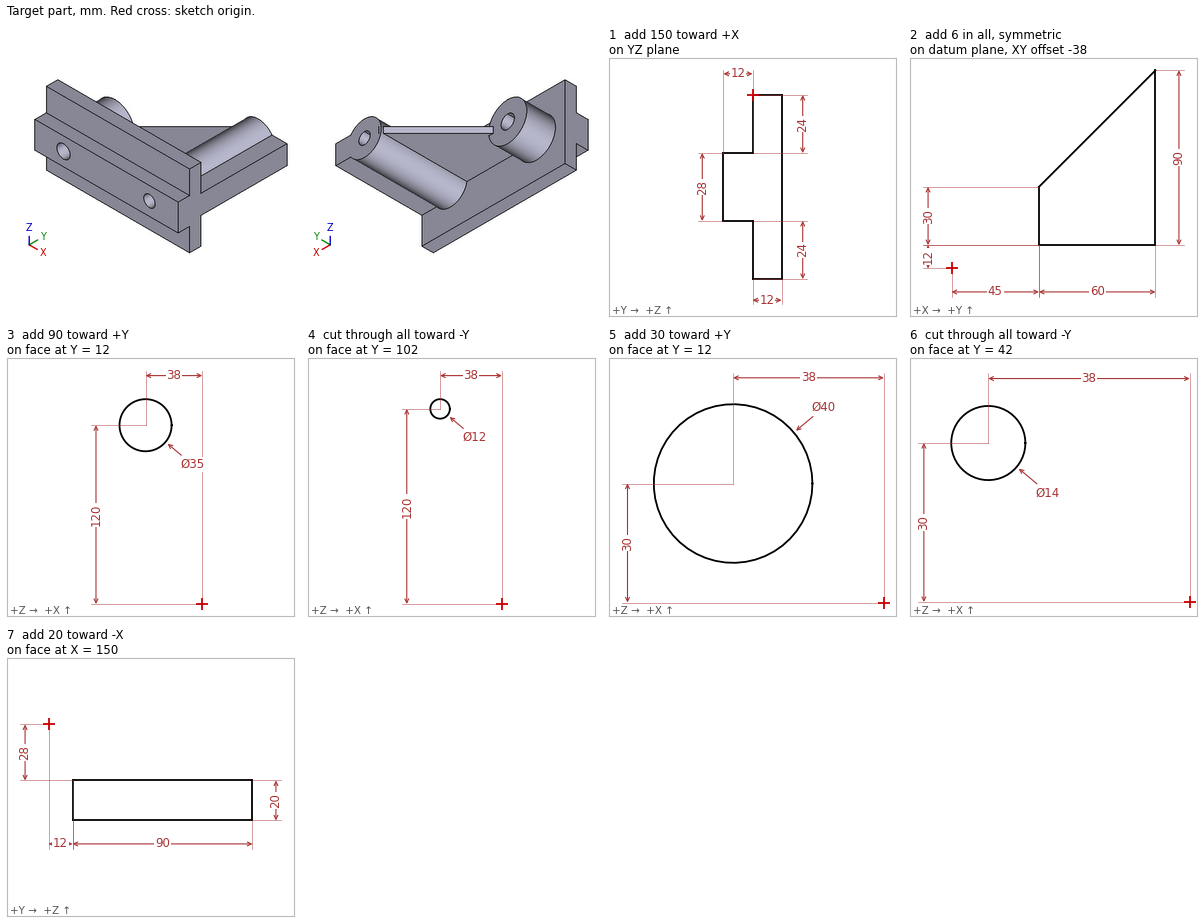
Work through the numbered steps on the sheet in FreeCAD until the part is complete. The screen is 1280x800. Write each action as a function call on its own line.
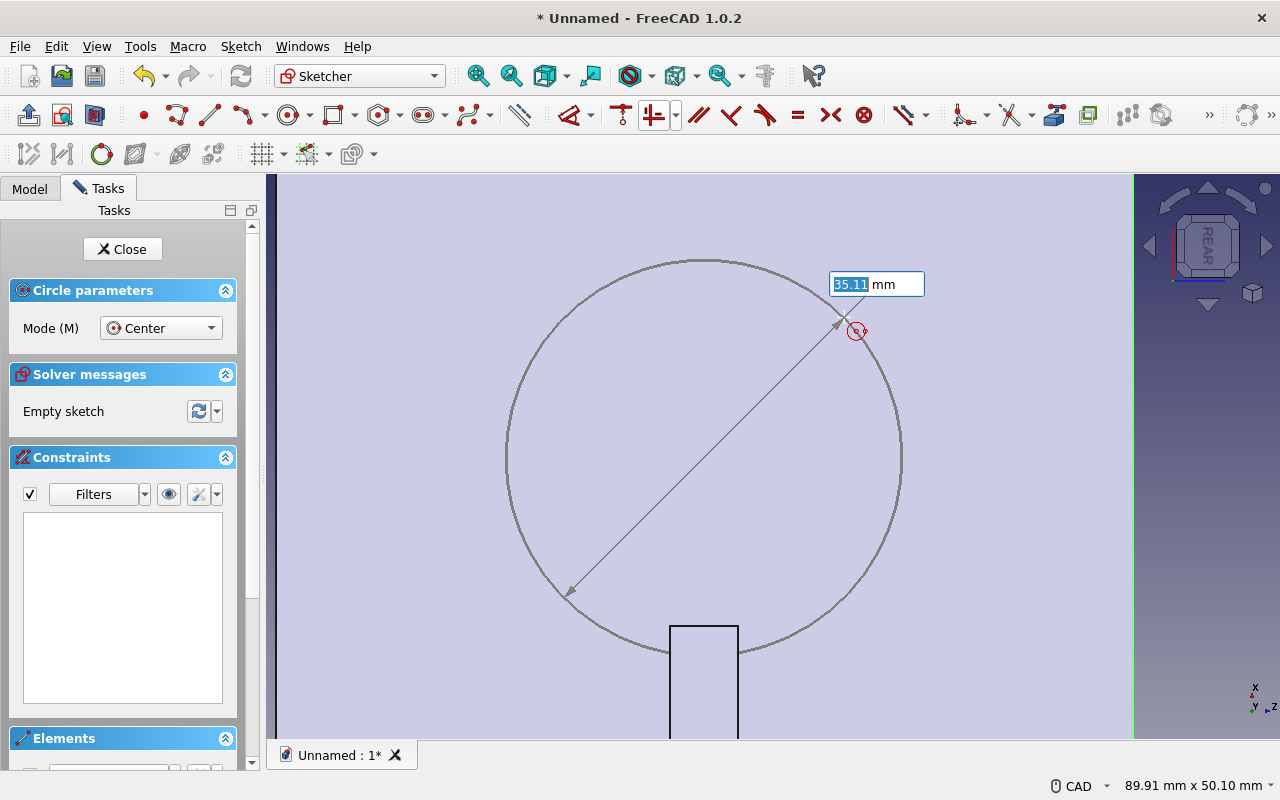
text(35)
key(Return)
key(Escape)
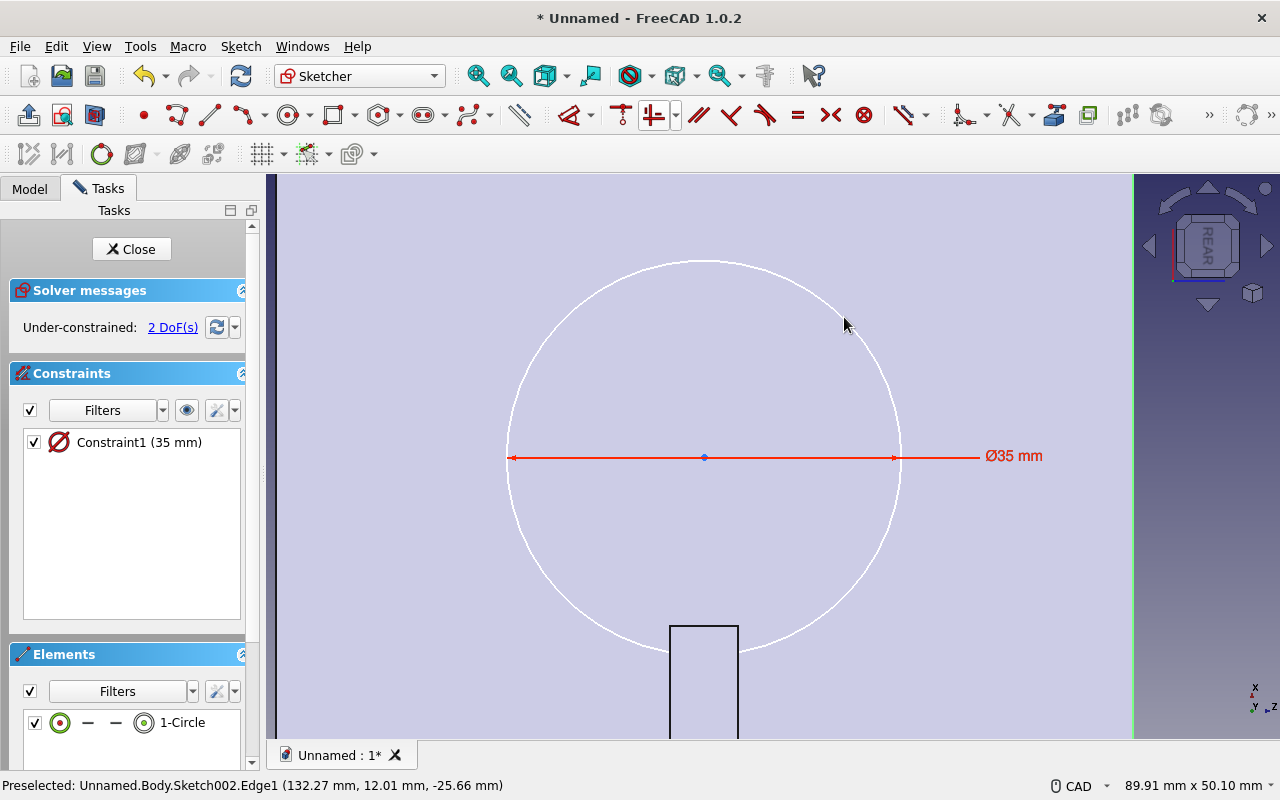
click(568, 116)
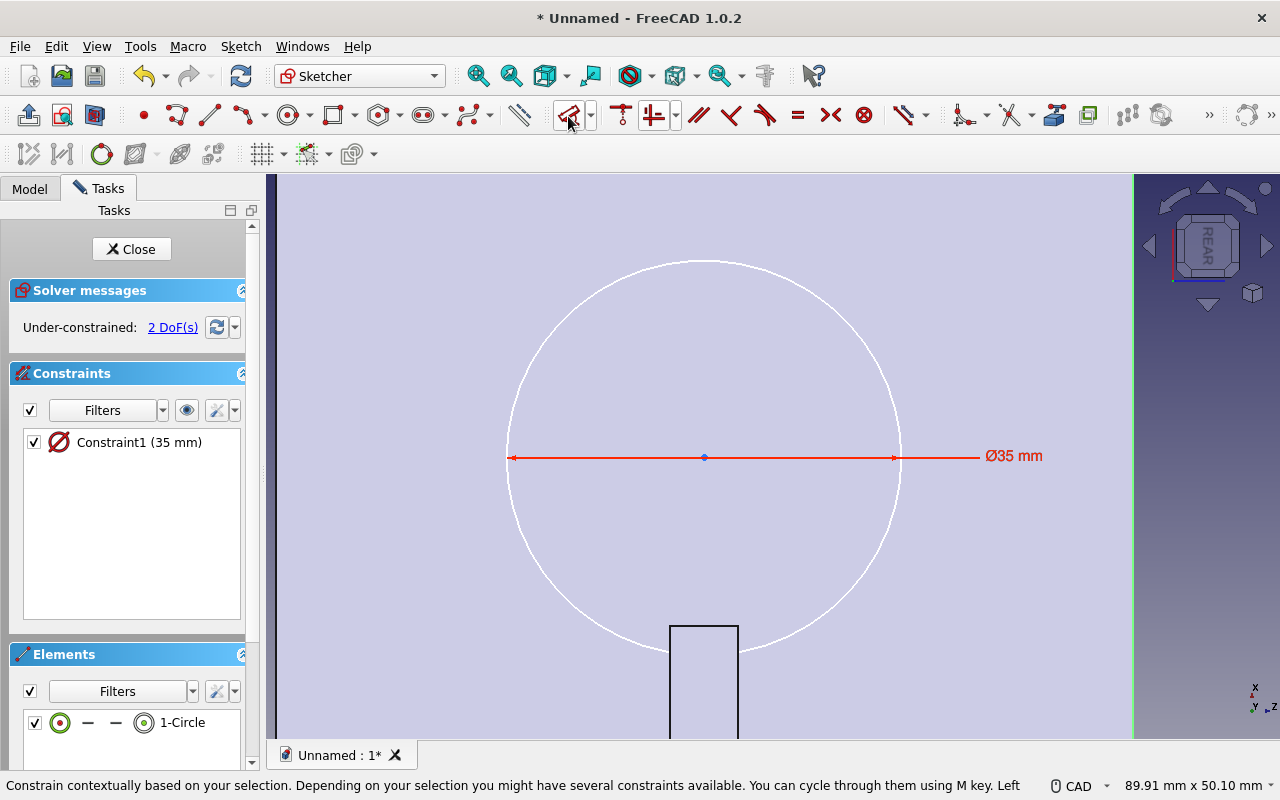
click(704, 458)
click(815, 424)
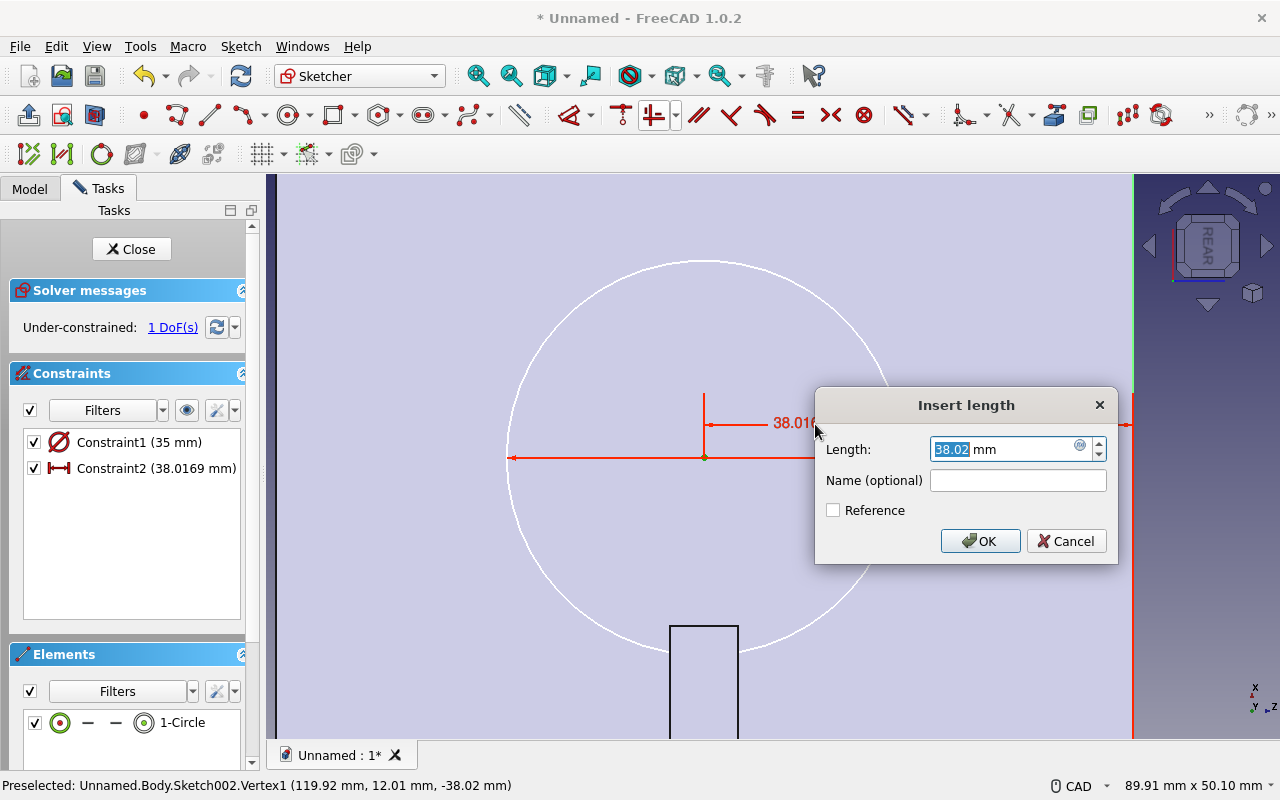
text(38)
key(Return)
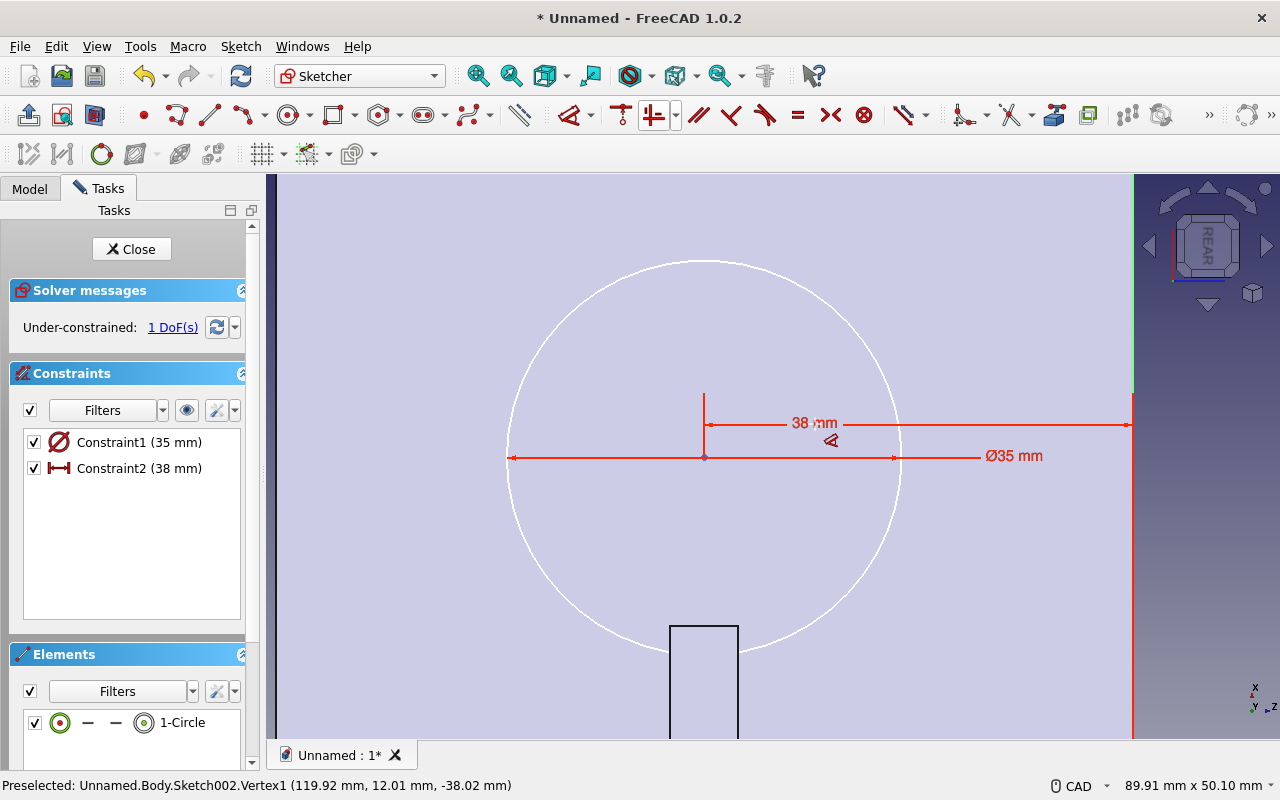
click(704, 458)
click(670, 585)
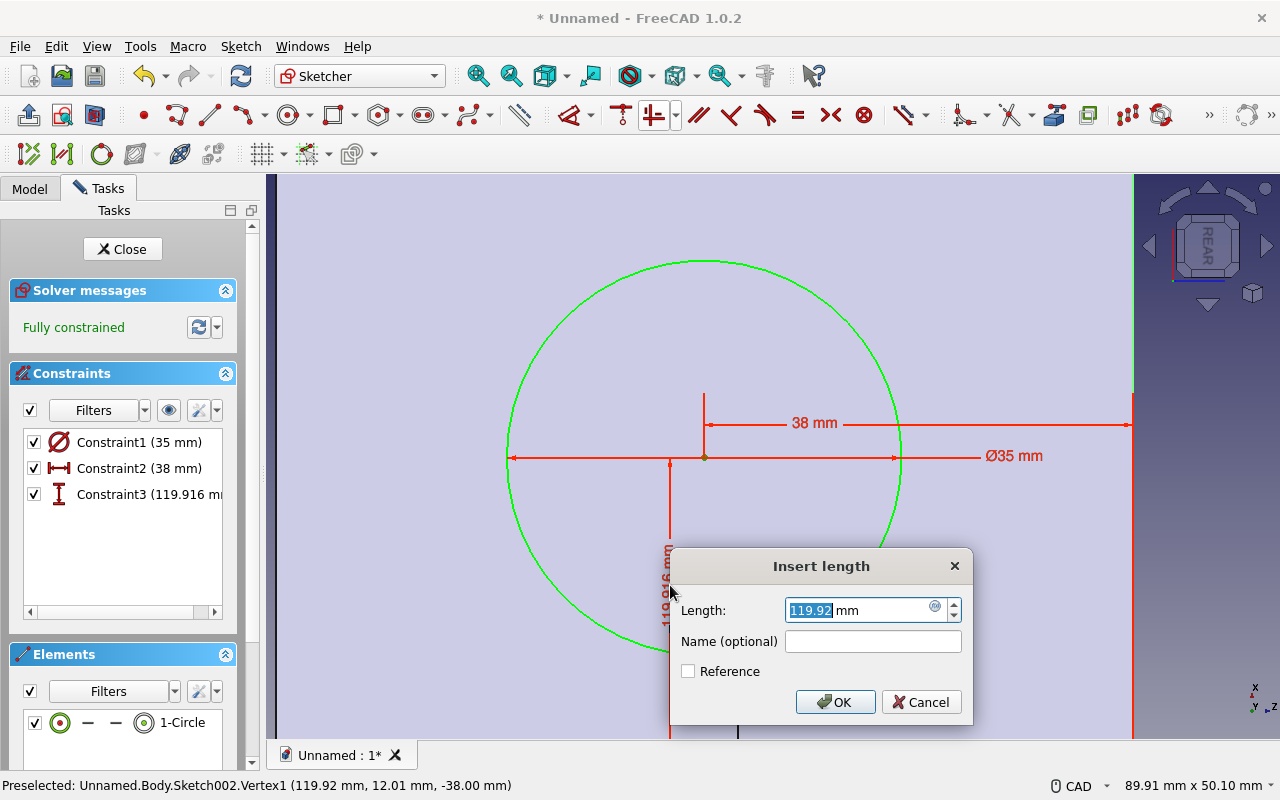
text(120)
key(Return)
key(Escape)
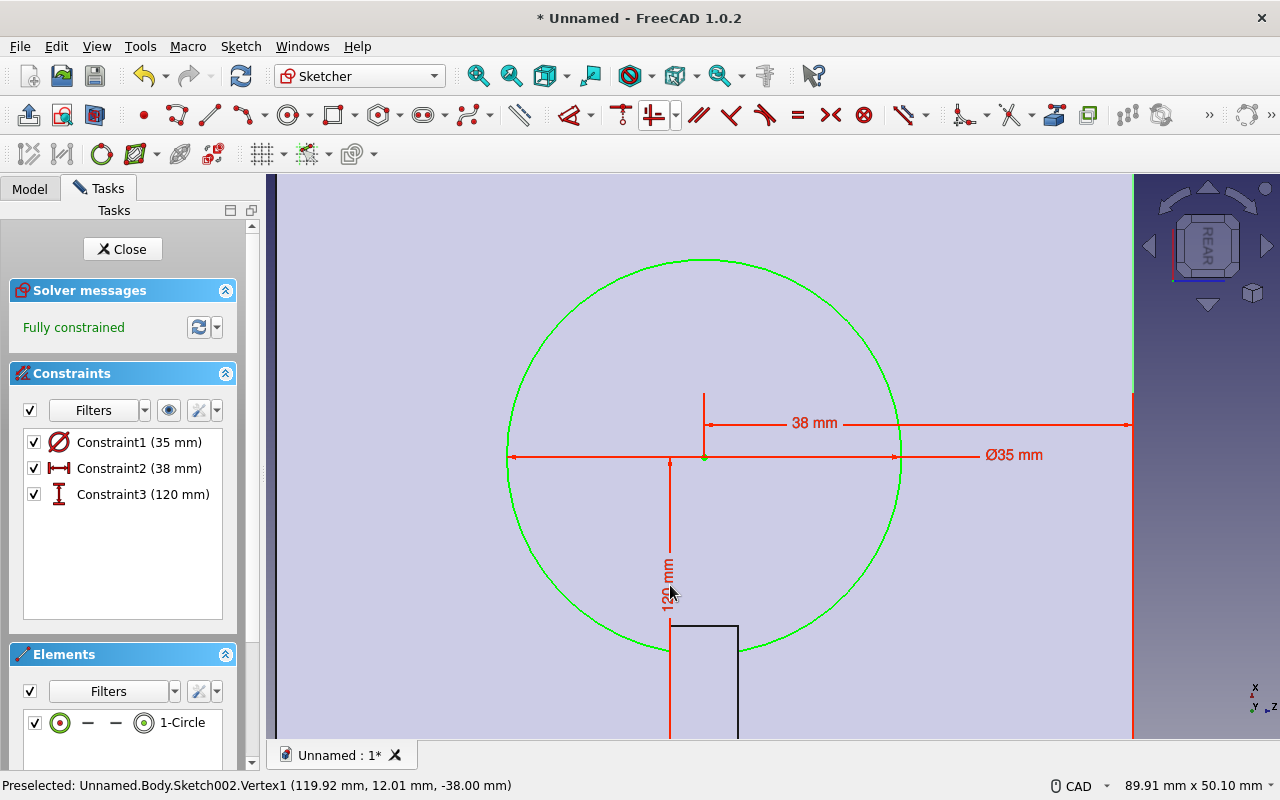
click(123, 249)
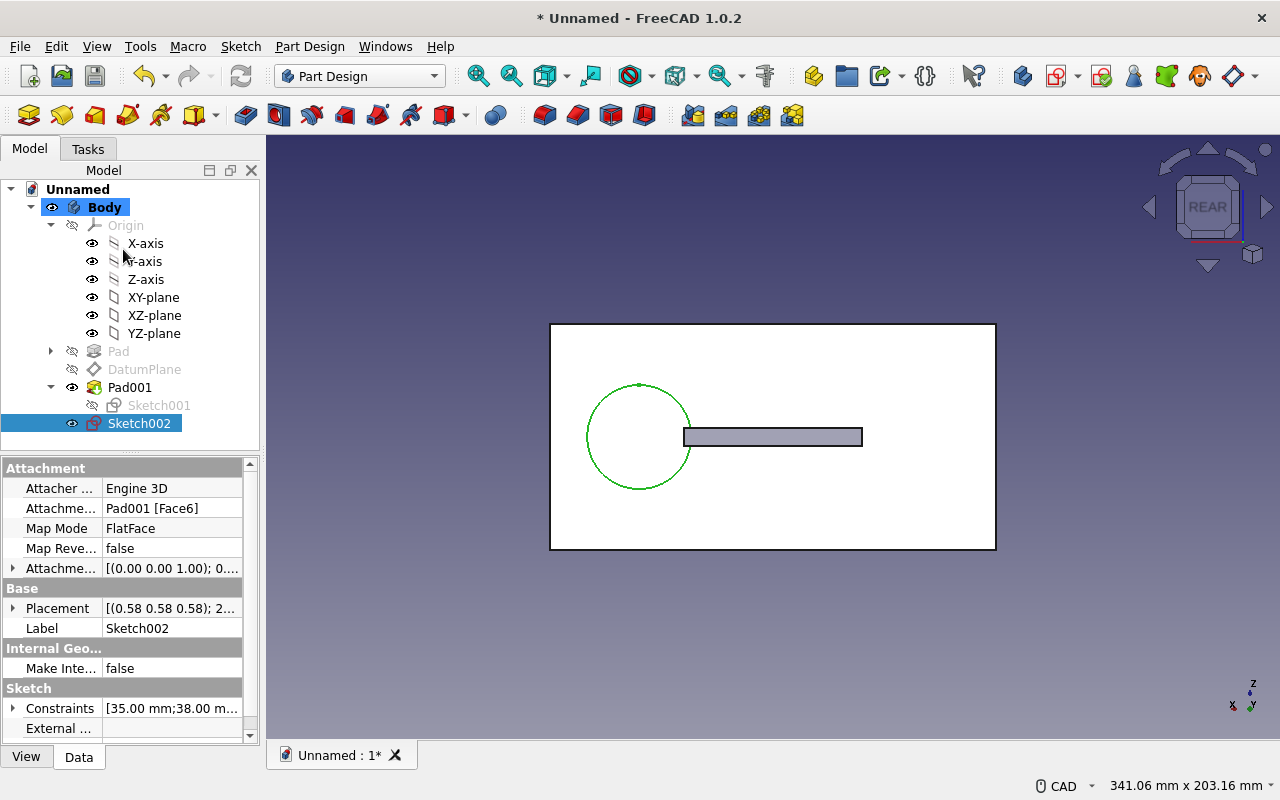
click(29, 116)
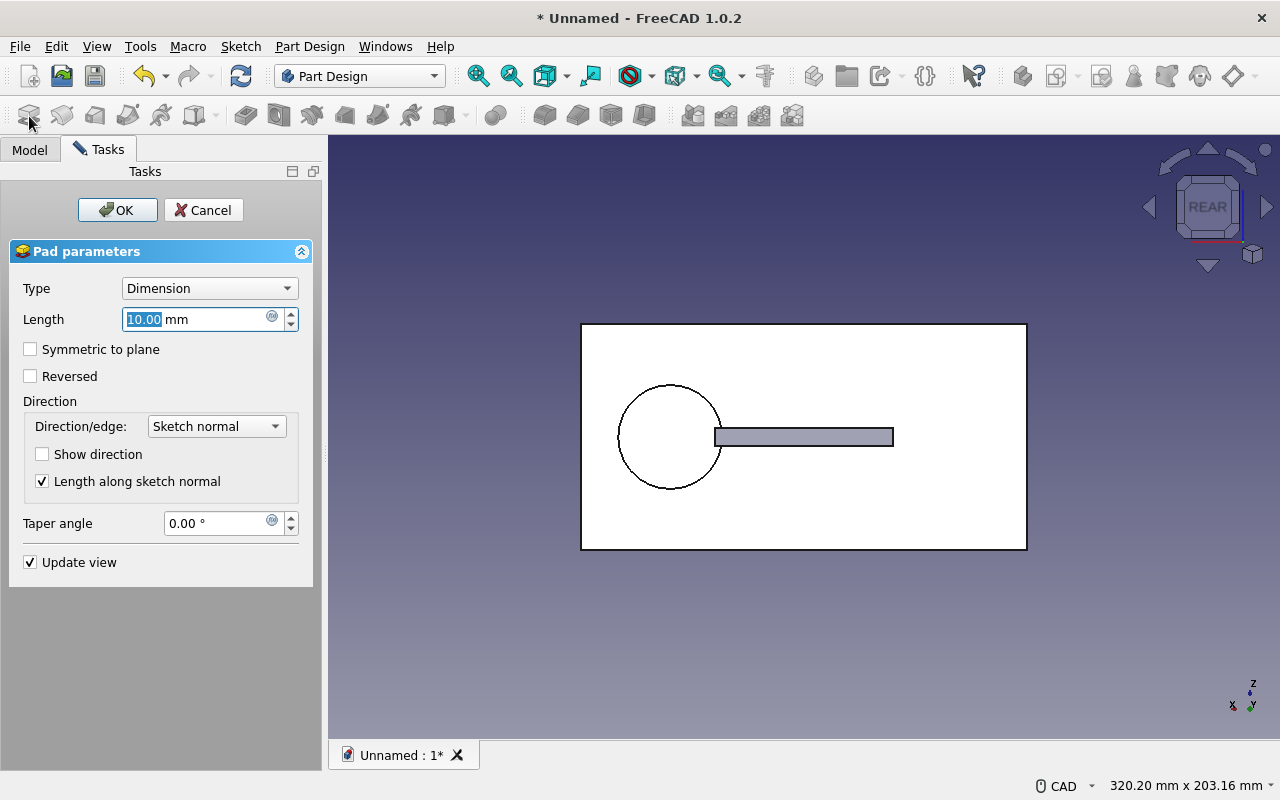
text(90)
key(Tab)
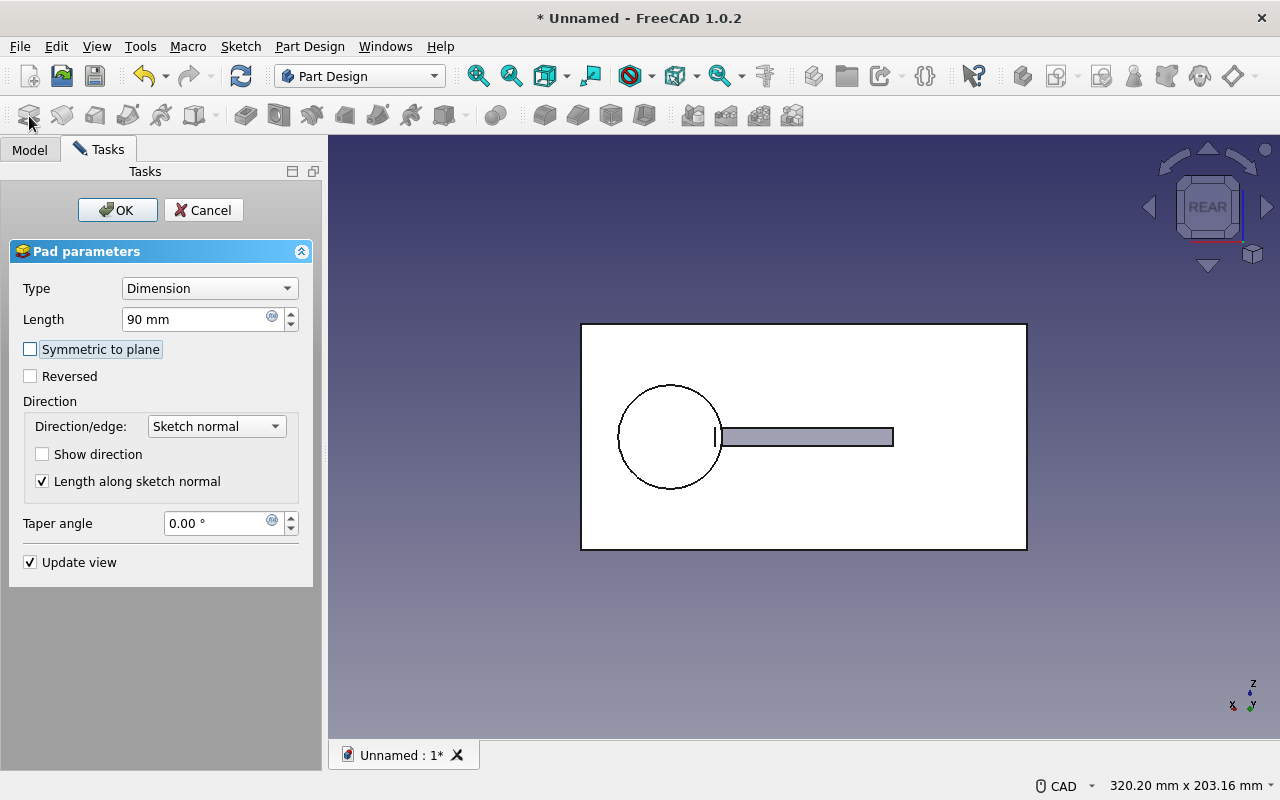
click(118, 210)